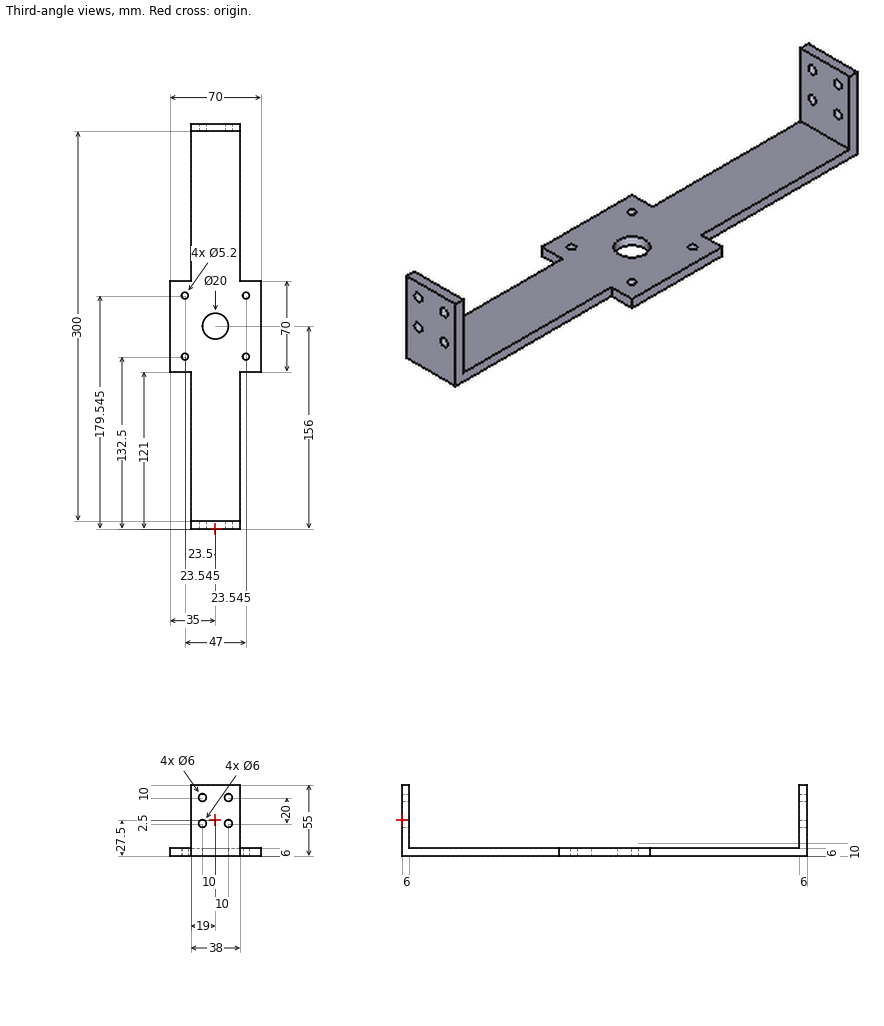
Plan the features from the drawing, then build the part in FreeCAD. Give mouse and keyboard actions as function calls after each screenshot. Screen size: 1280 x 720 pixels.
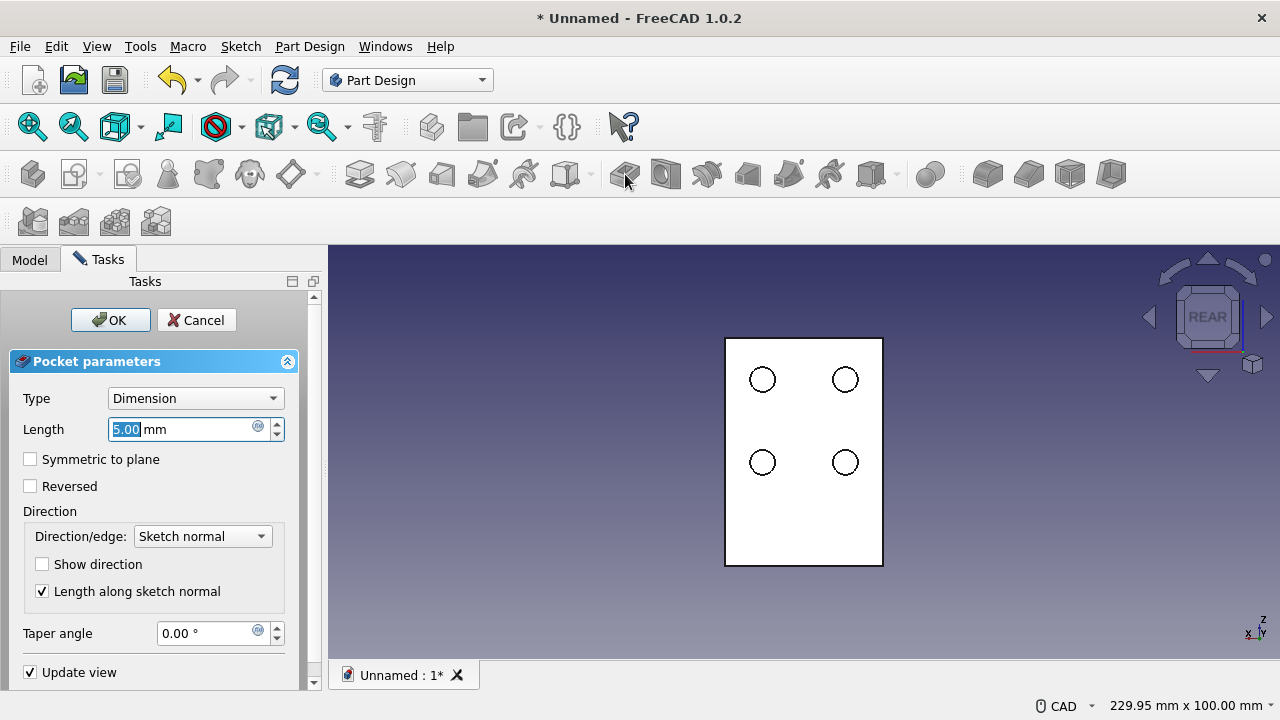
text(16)
key(Tab)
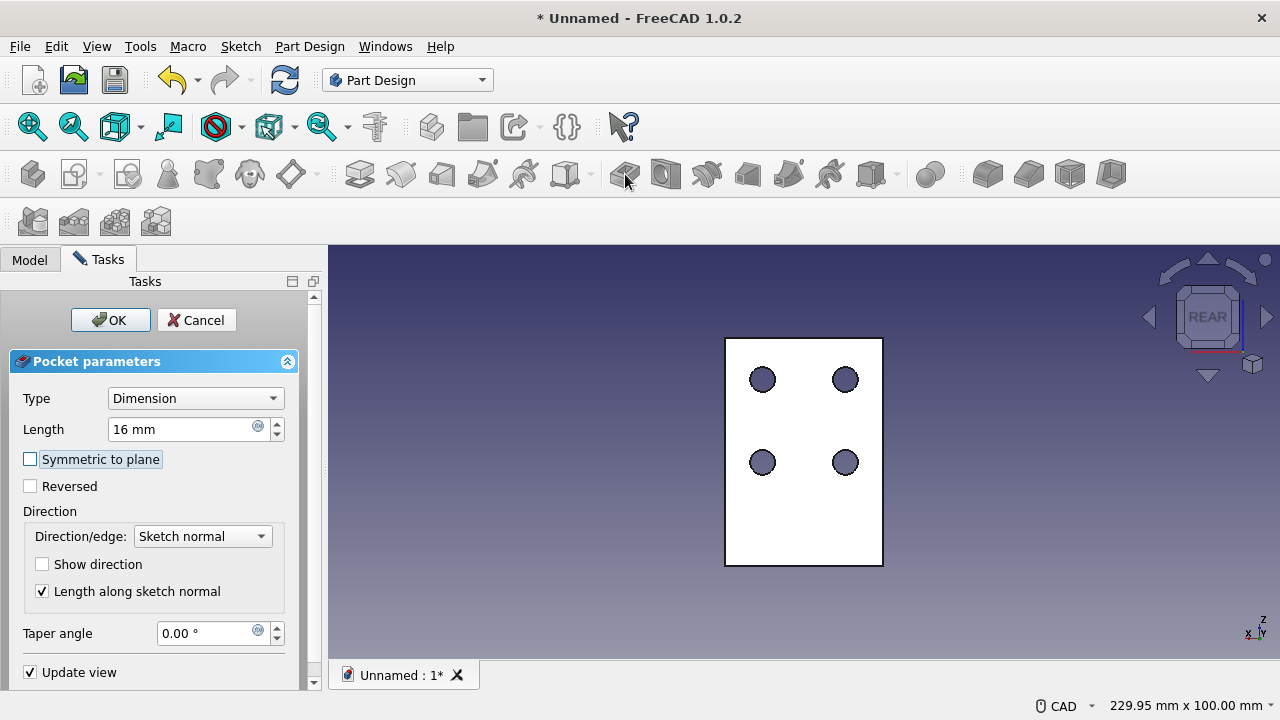
click(111, 320)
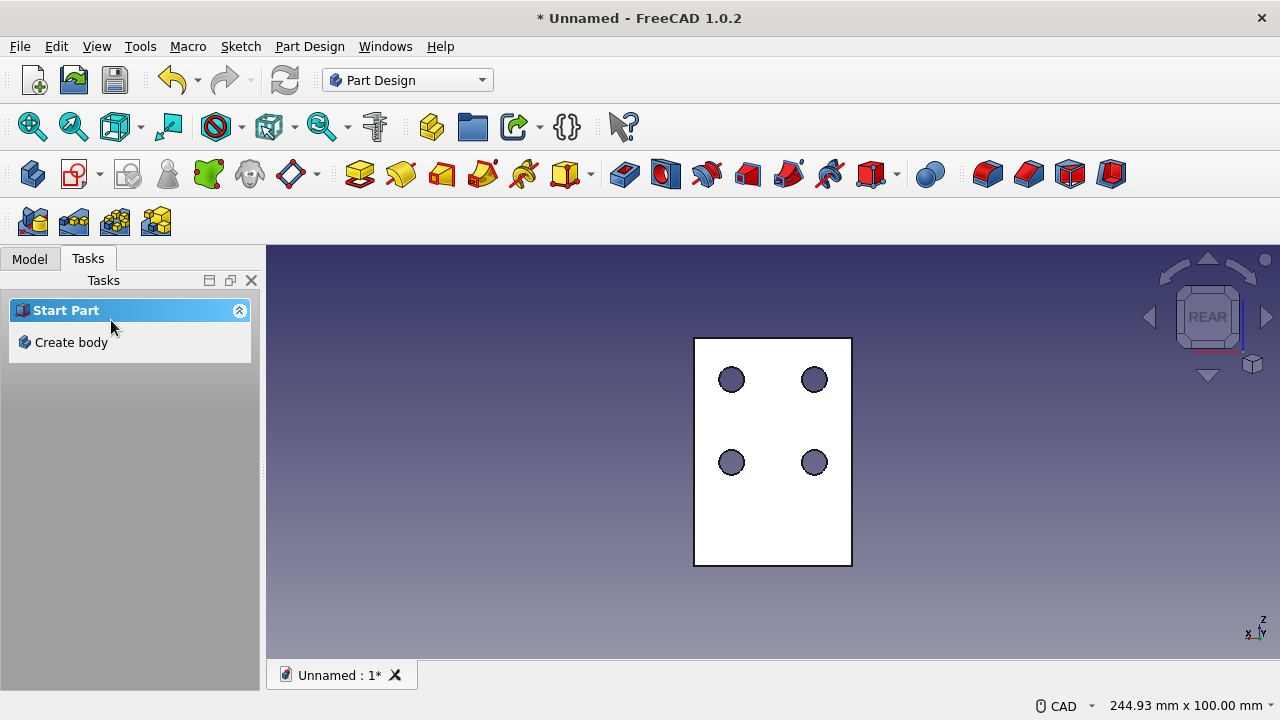
click(773, 516)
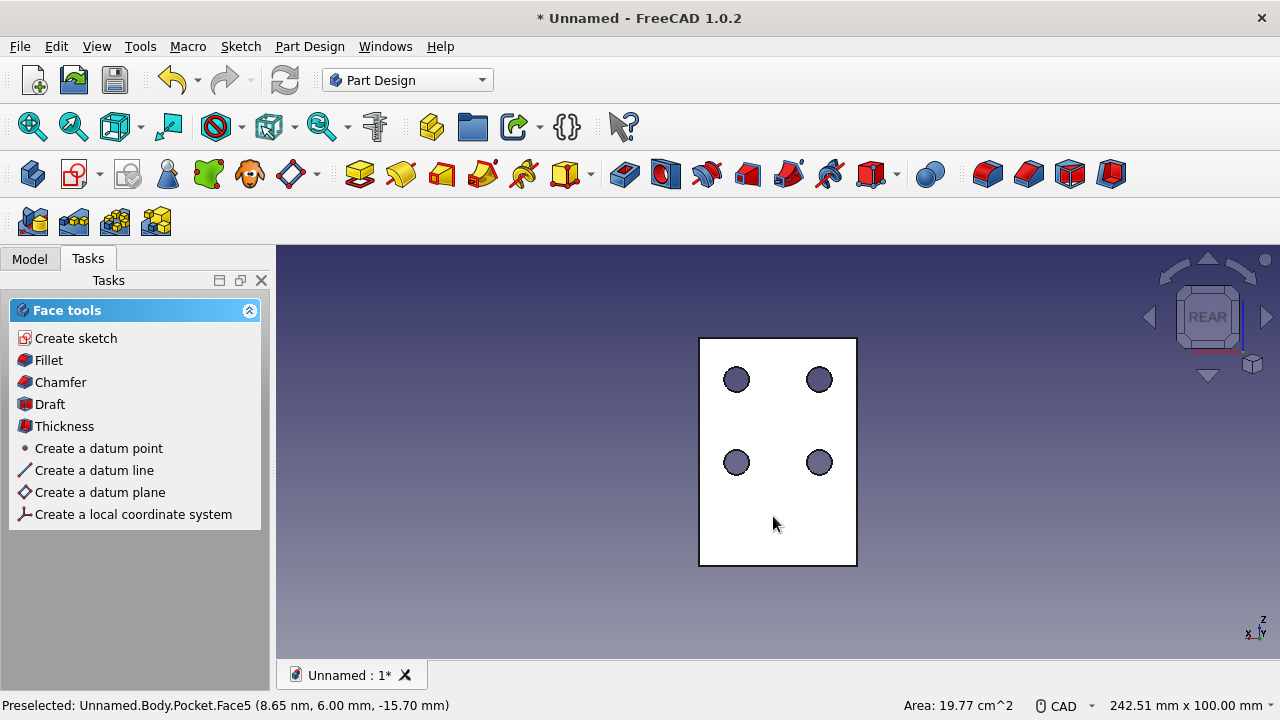
click(74, 174)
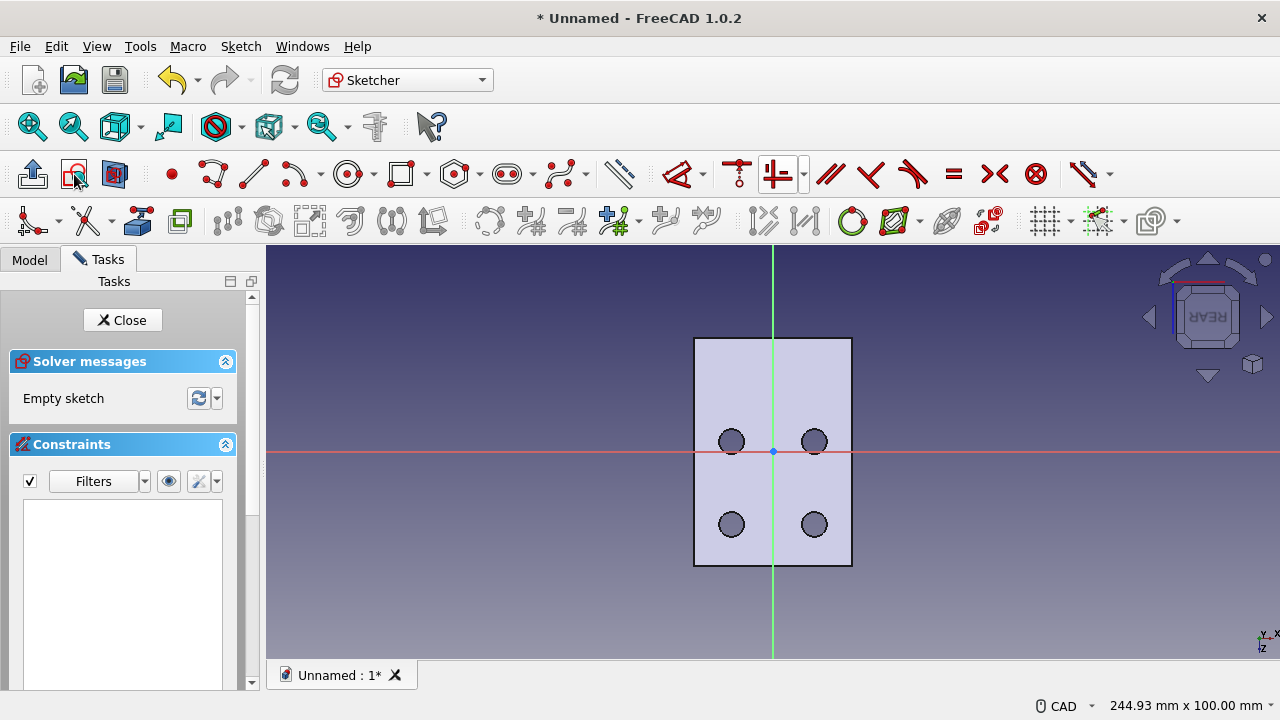
scroll(829, 349, up, 4)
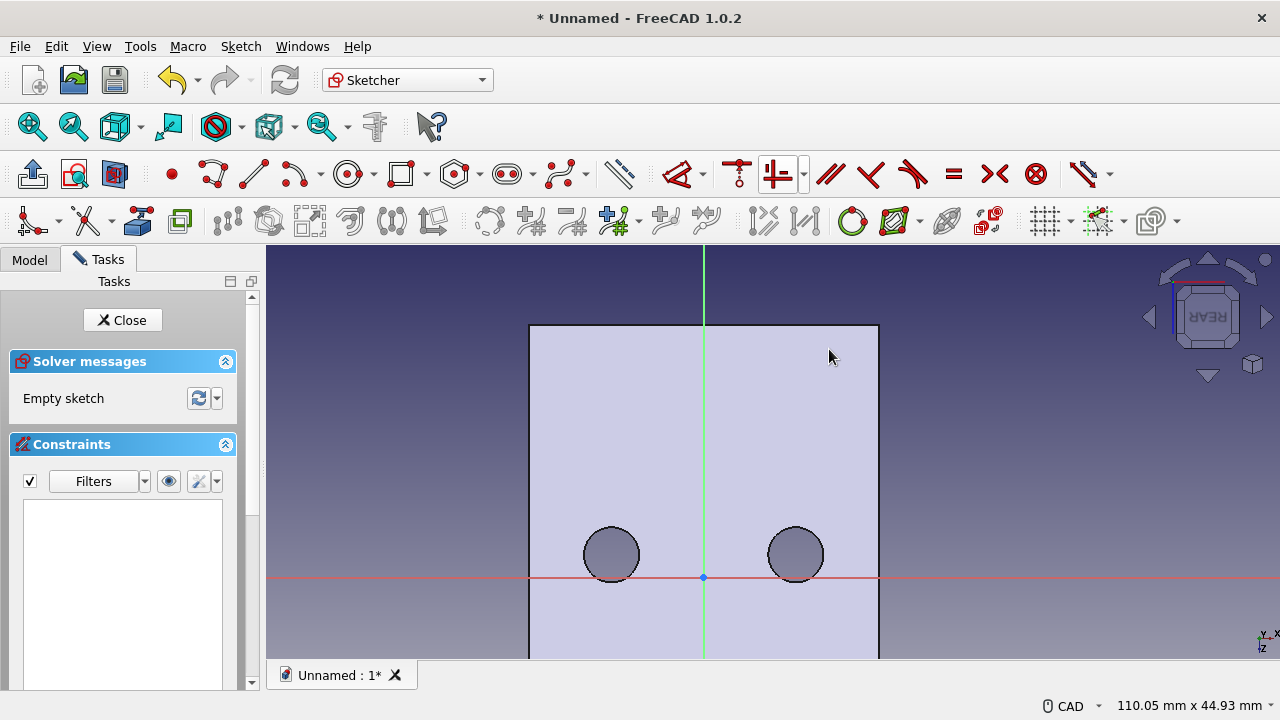
click(400, 174)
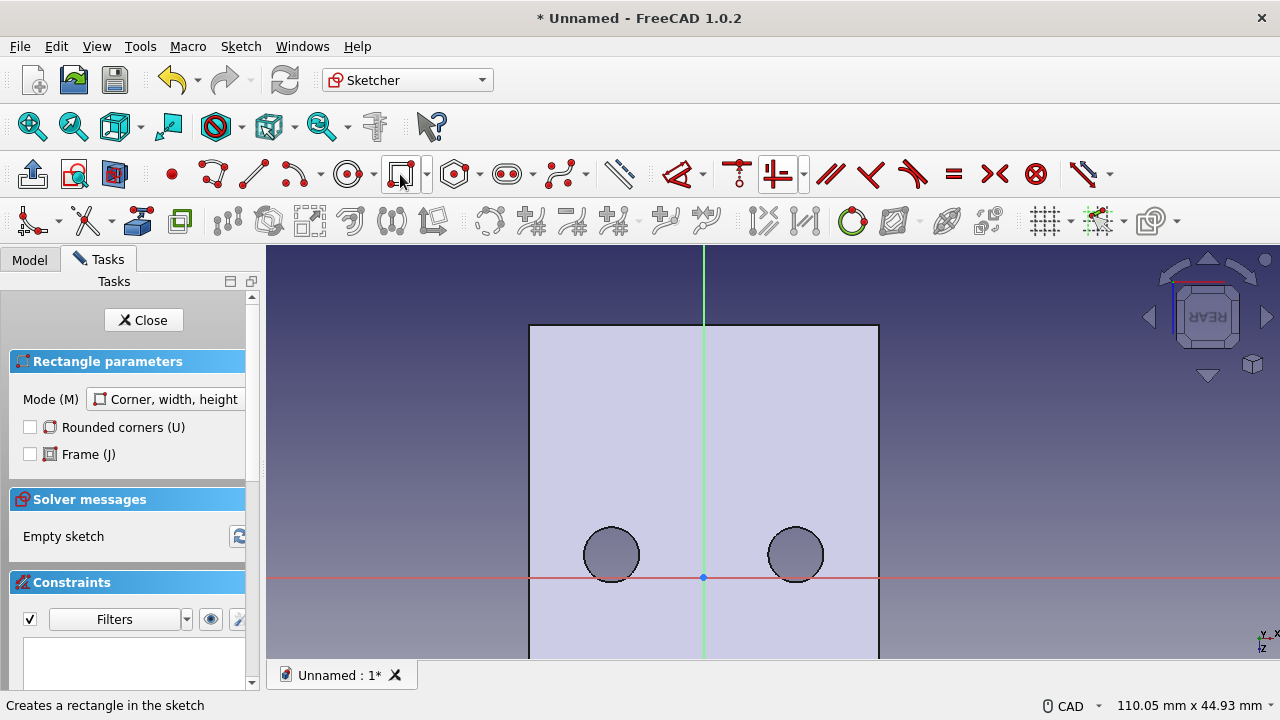
click(529, 325)
move(879, 380)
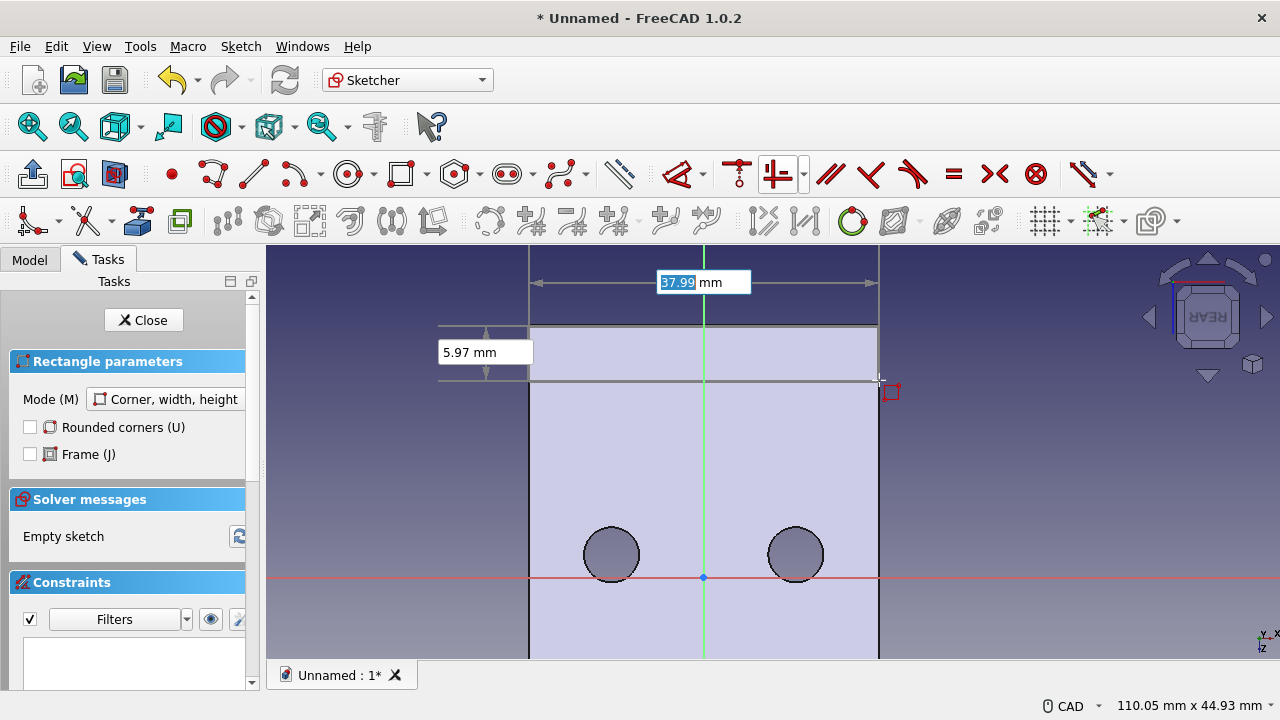
text(38)
key(Tab)
text(6)
key(Return)
key(Escape)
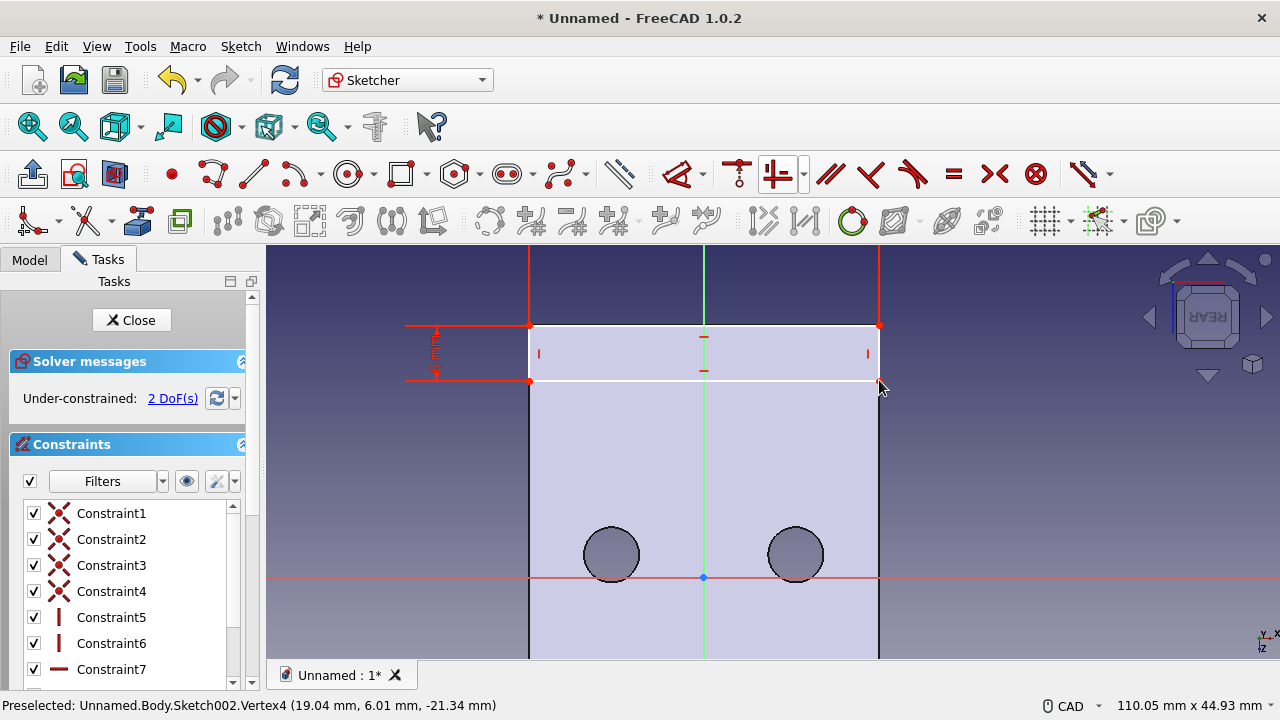
key(d)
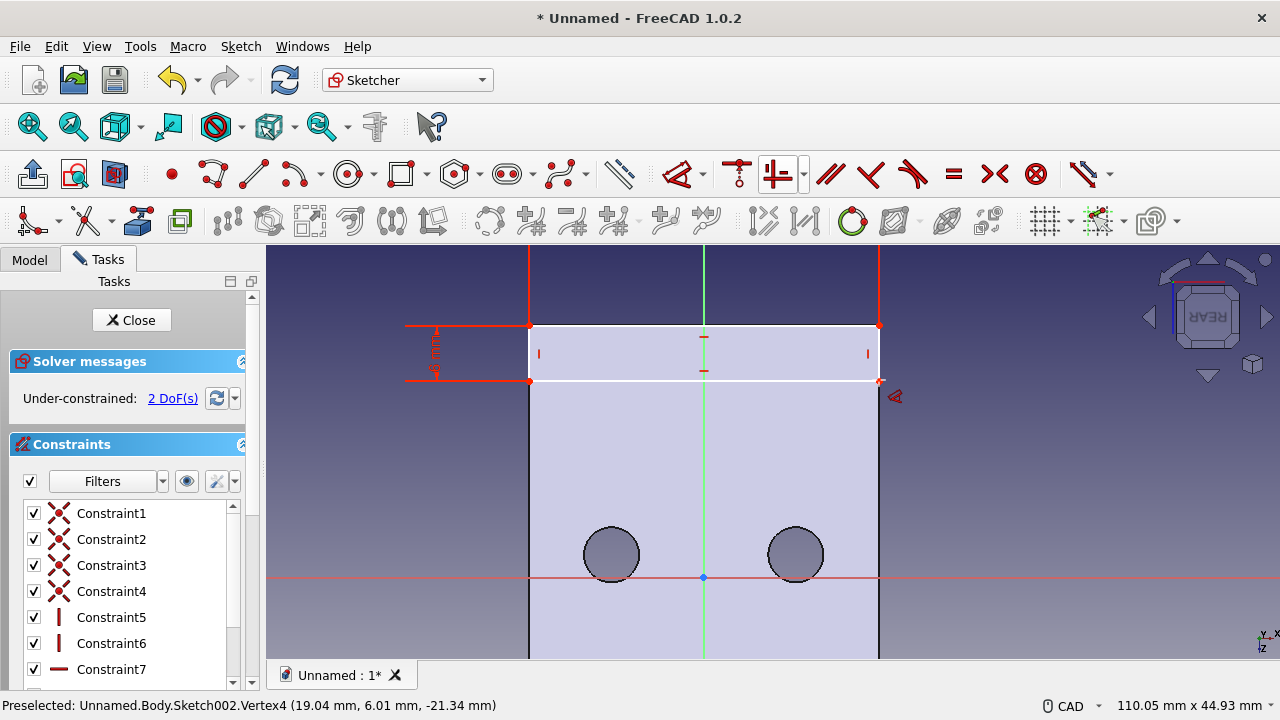
click(529, 326)
click(616, 612)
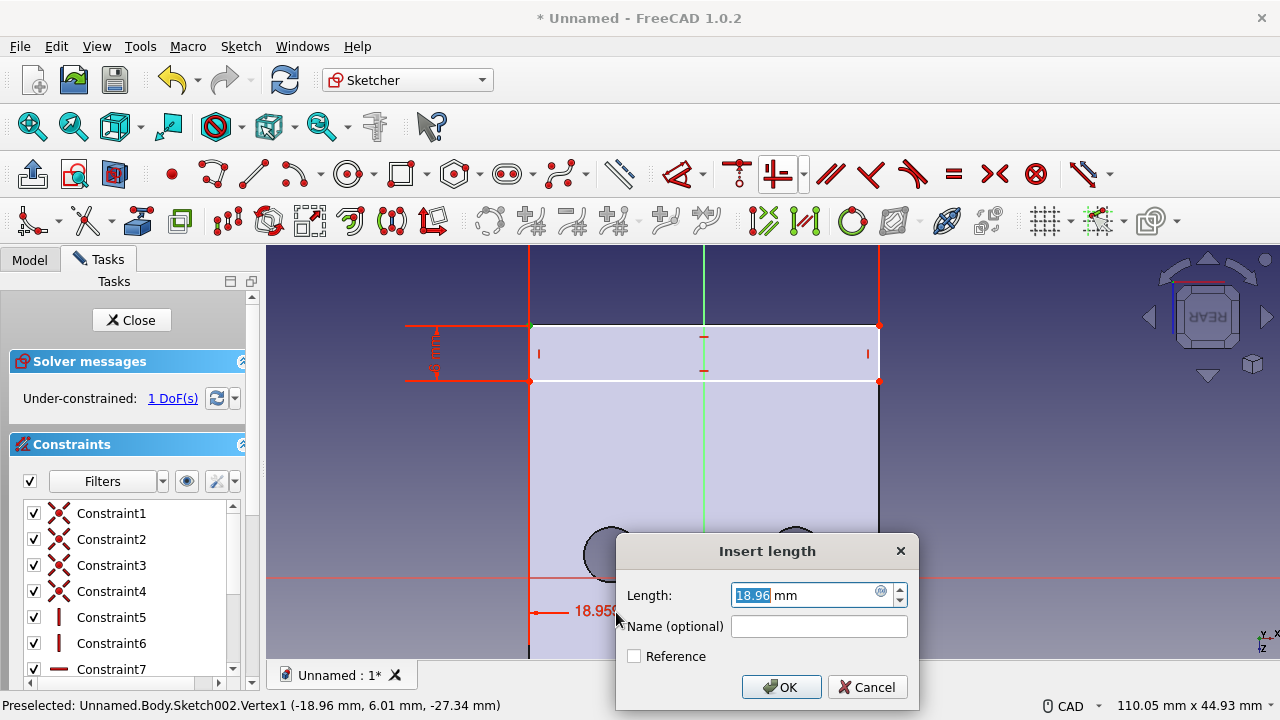
text(19)
key(Return)